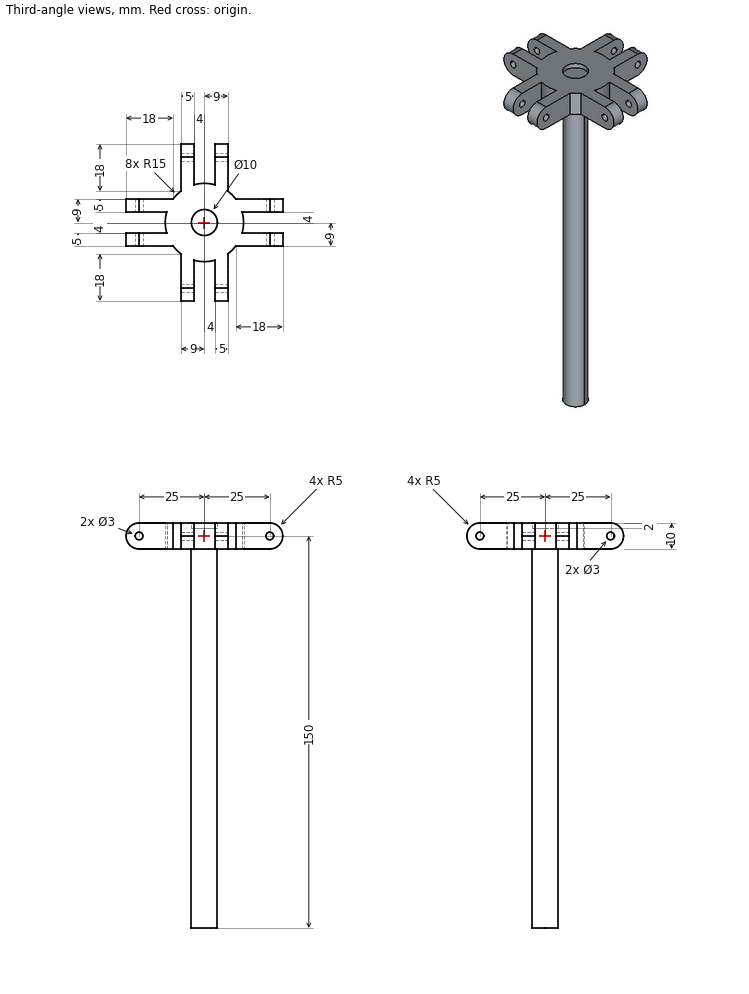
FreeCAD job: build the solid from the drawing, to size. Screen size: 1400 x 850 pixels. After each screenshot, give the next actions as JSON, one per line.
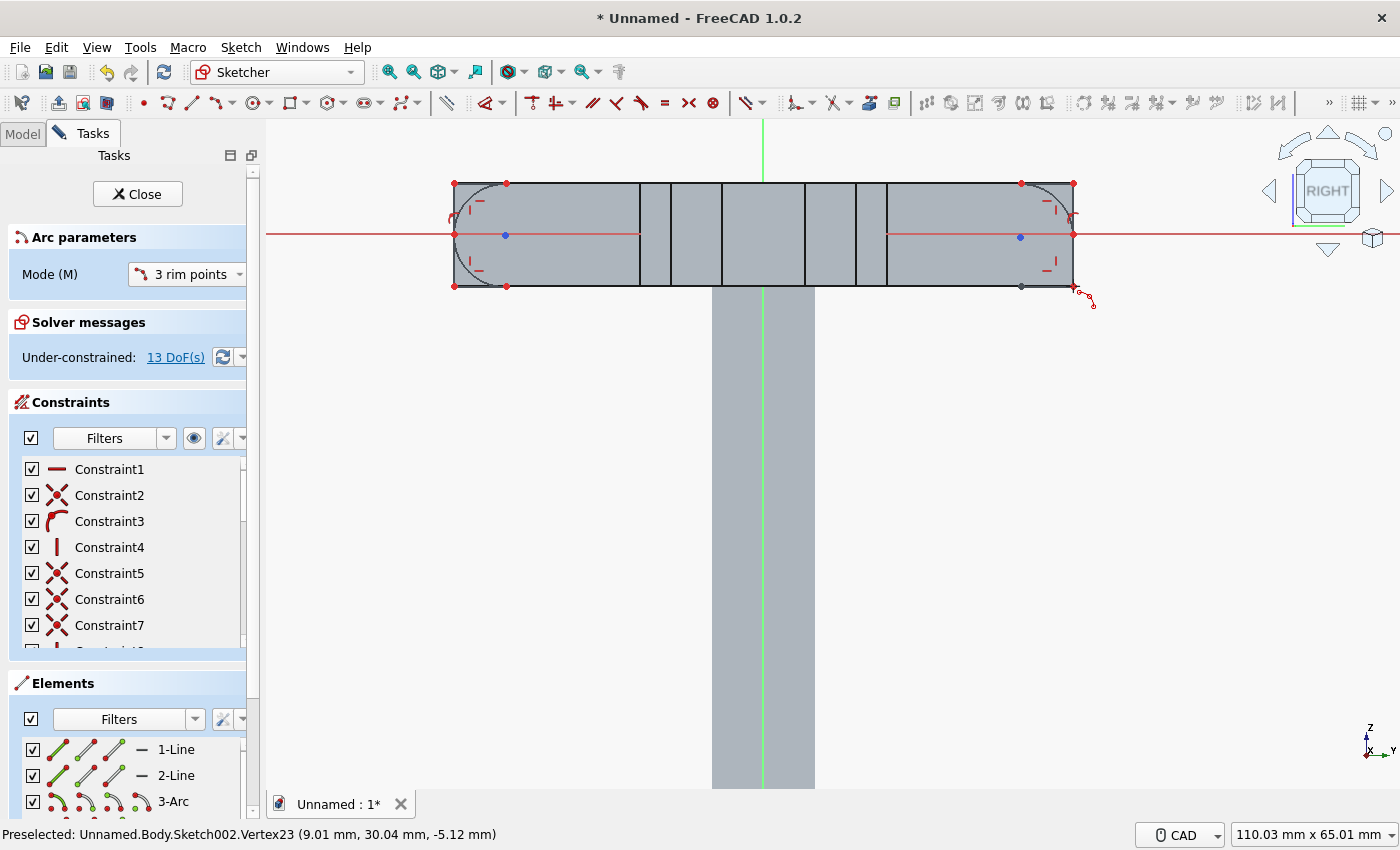
{"action": "left_click", "coordinate": [1073, 234]}
{"action": "left_click", "coordinate": [1021, 287]}
{"action": "left_click", "coordinate": [1057, 271]}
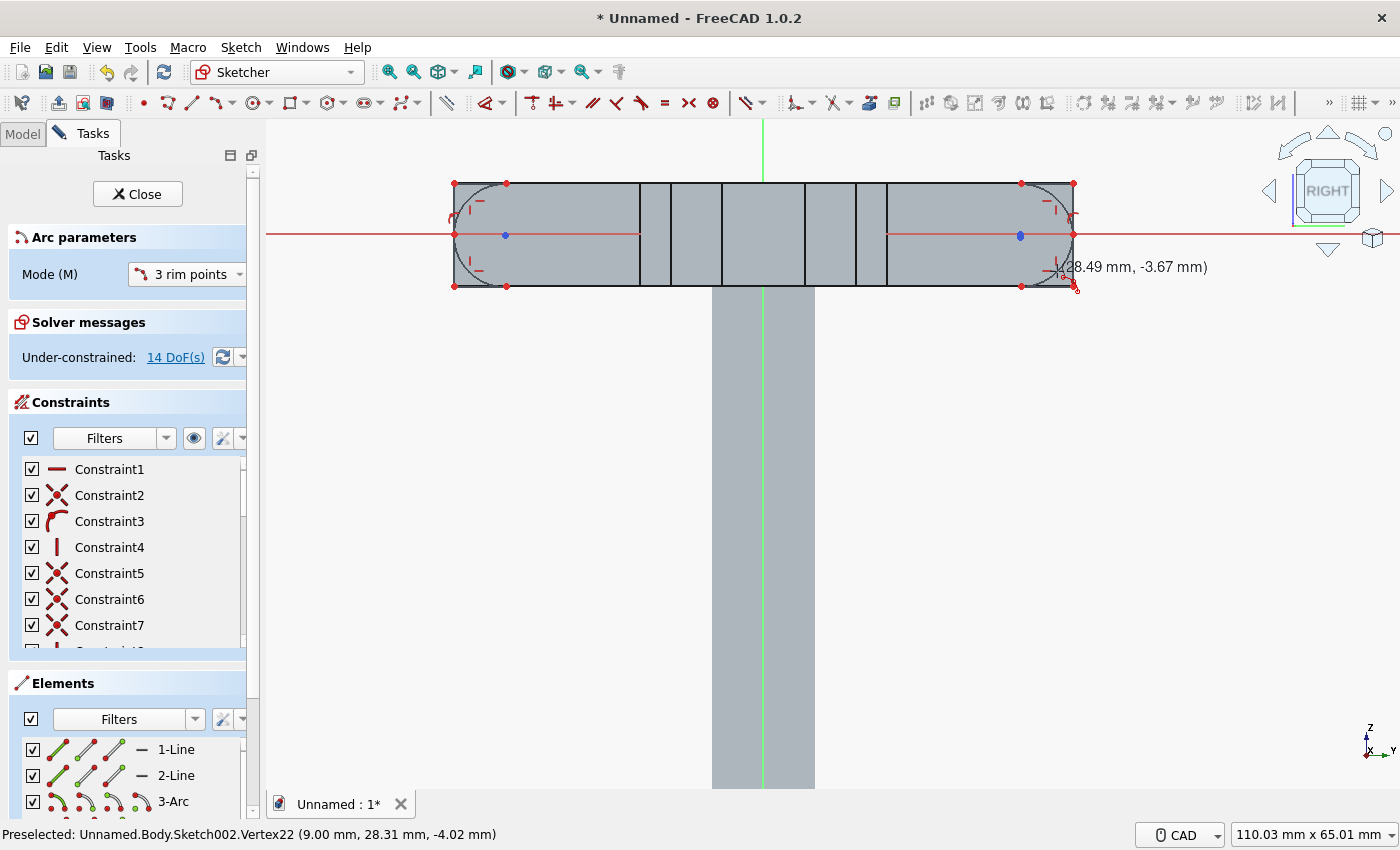
{"action": "key", "text": "g c"}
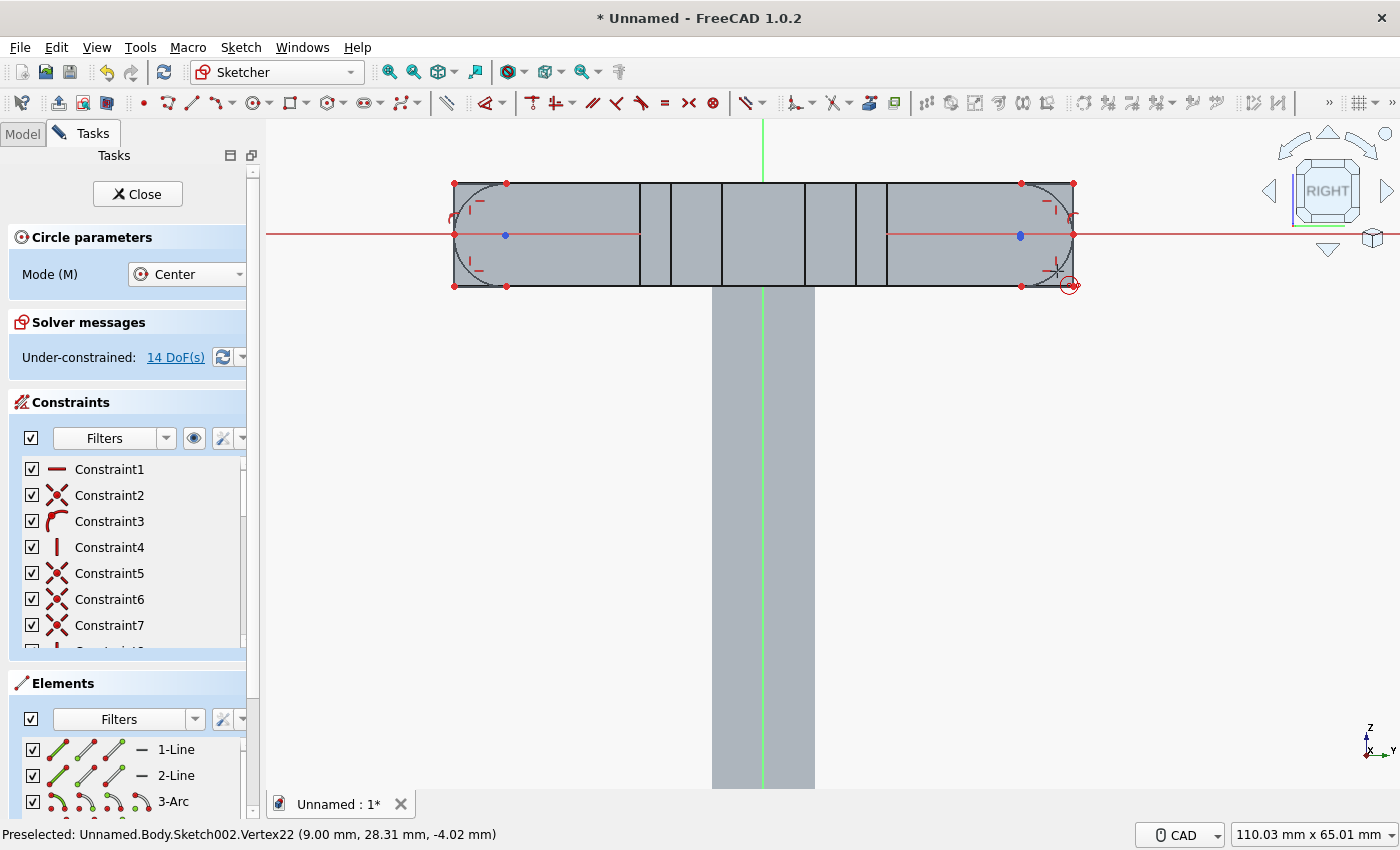
{"action": "scroll", "coordinate": [1021, 234], "scroll_direction": "up", "scroll_amount": 2}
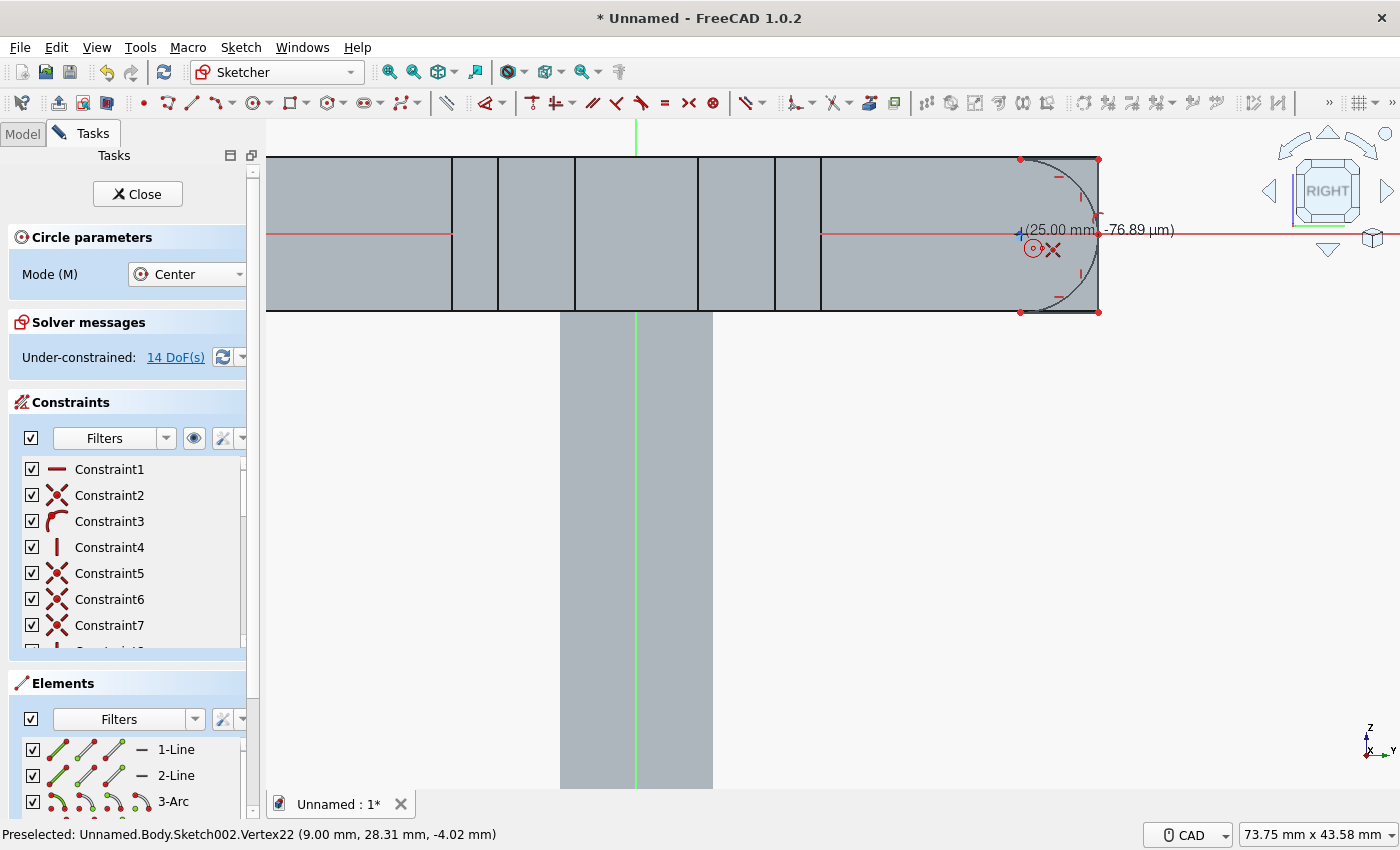
{"action": "left_click", "coordinate": [1021, 234]}
{"action": "mouse_move", "coordinate": [1037, 218]}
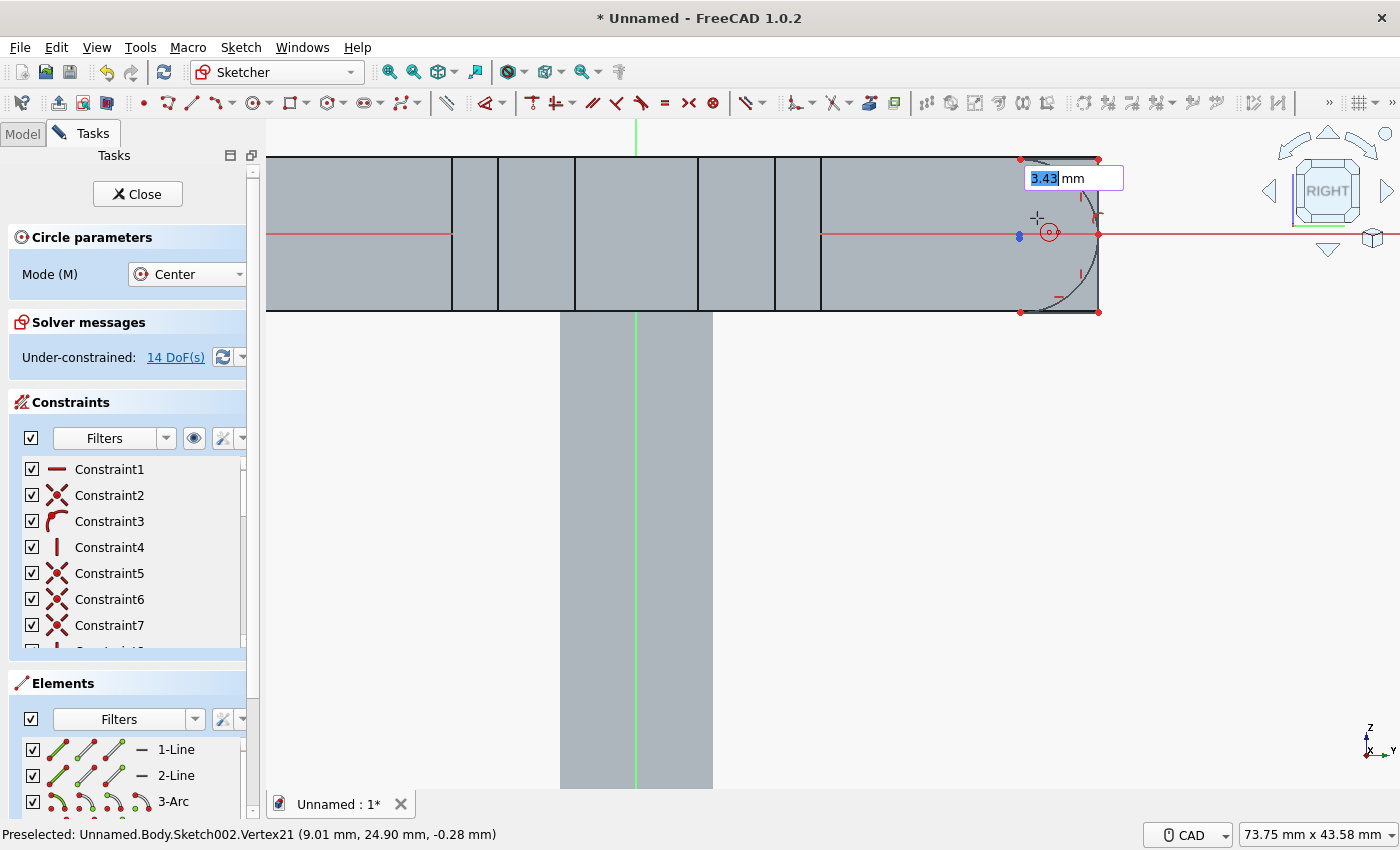
{"action": "type", "text": "3"}
{"action": "key", "text": "Return"}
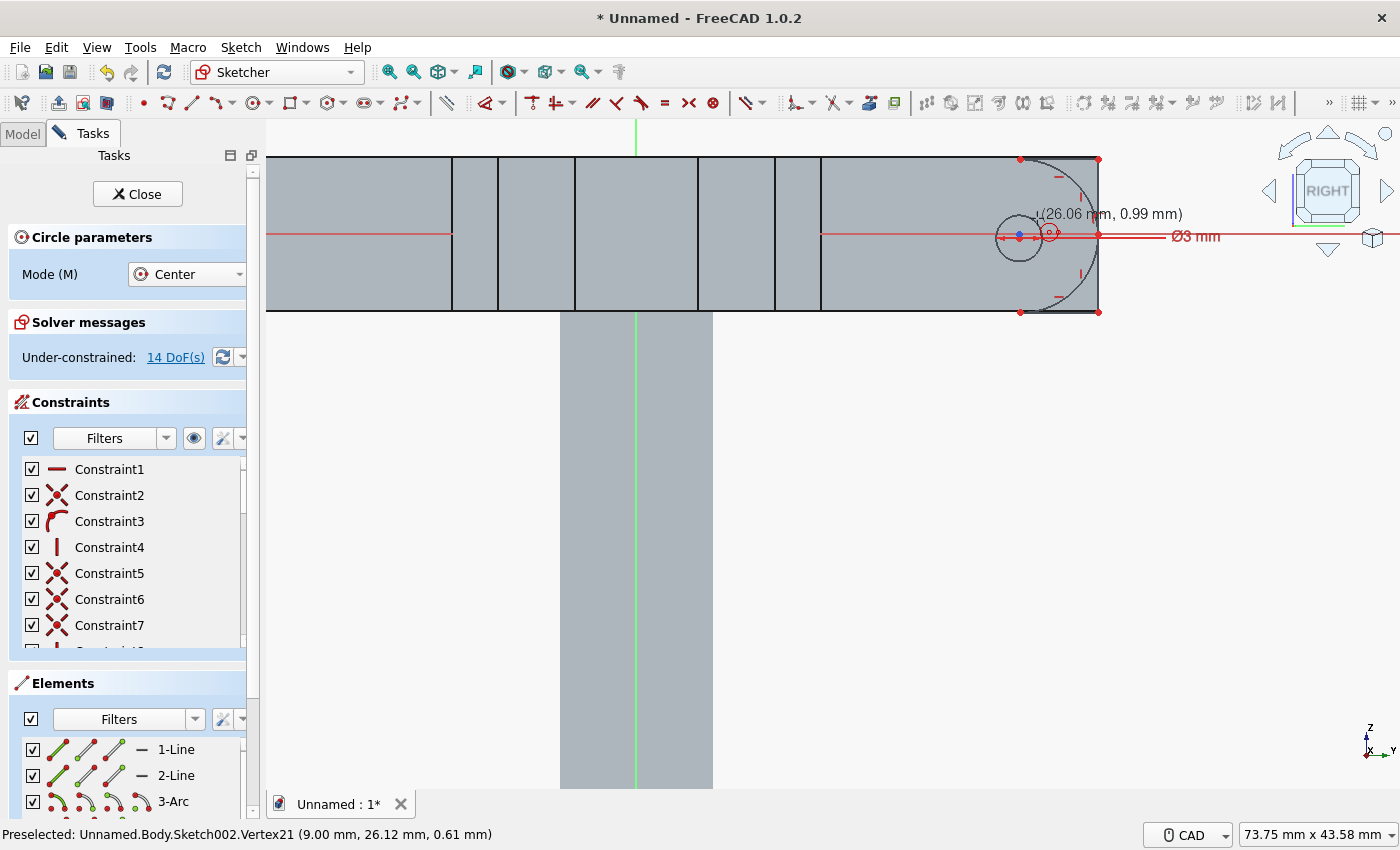
{"action": "scroll", "coordinate": [1025, 761], "scroll_direction": "down", "scroll_amount": 2}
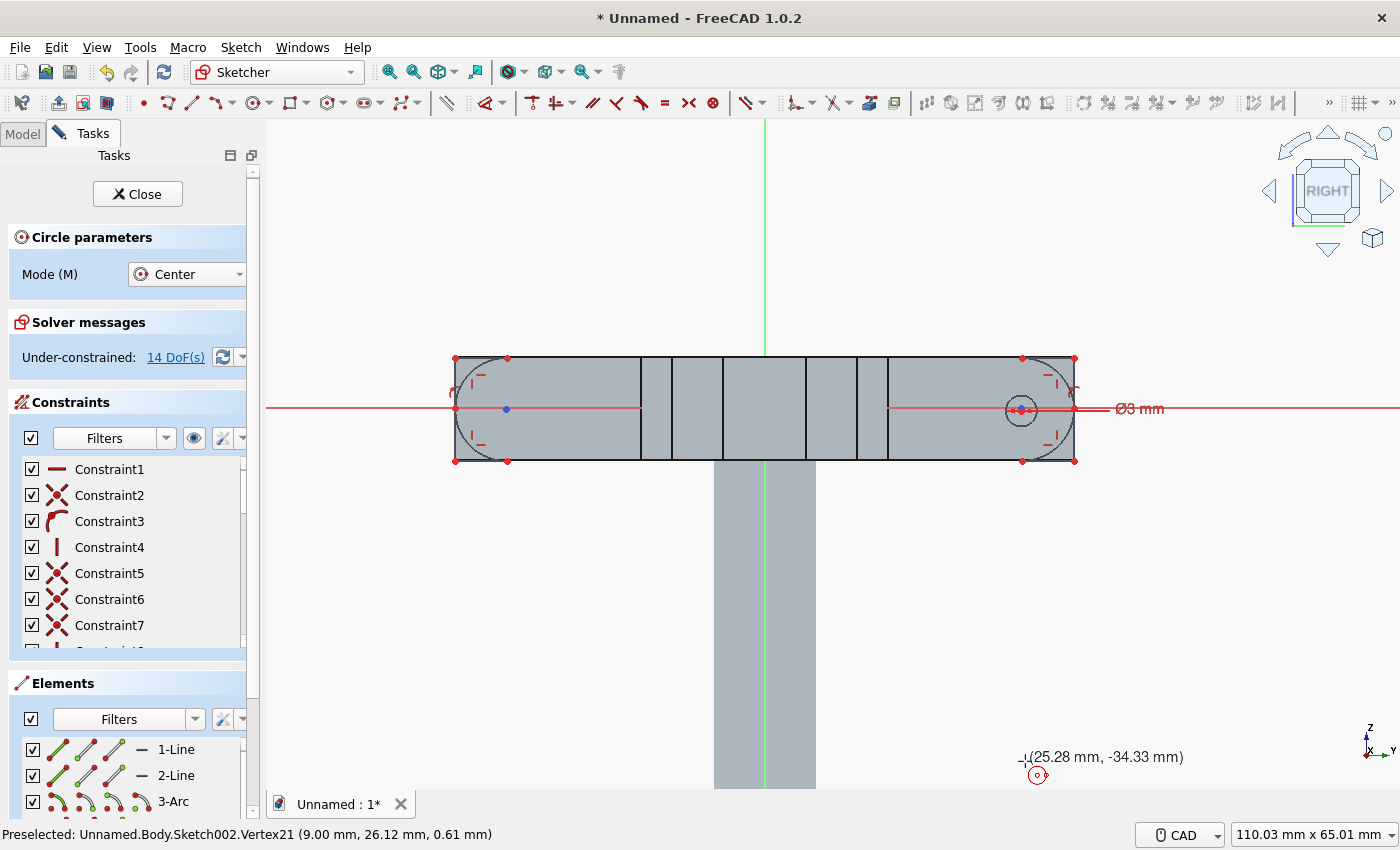
{"action": "scroll", "coordinate": [507, 408], "scroll_direction": "up", "scroll_amount": 2}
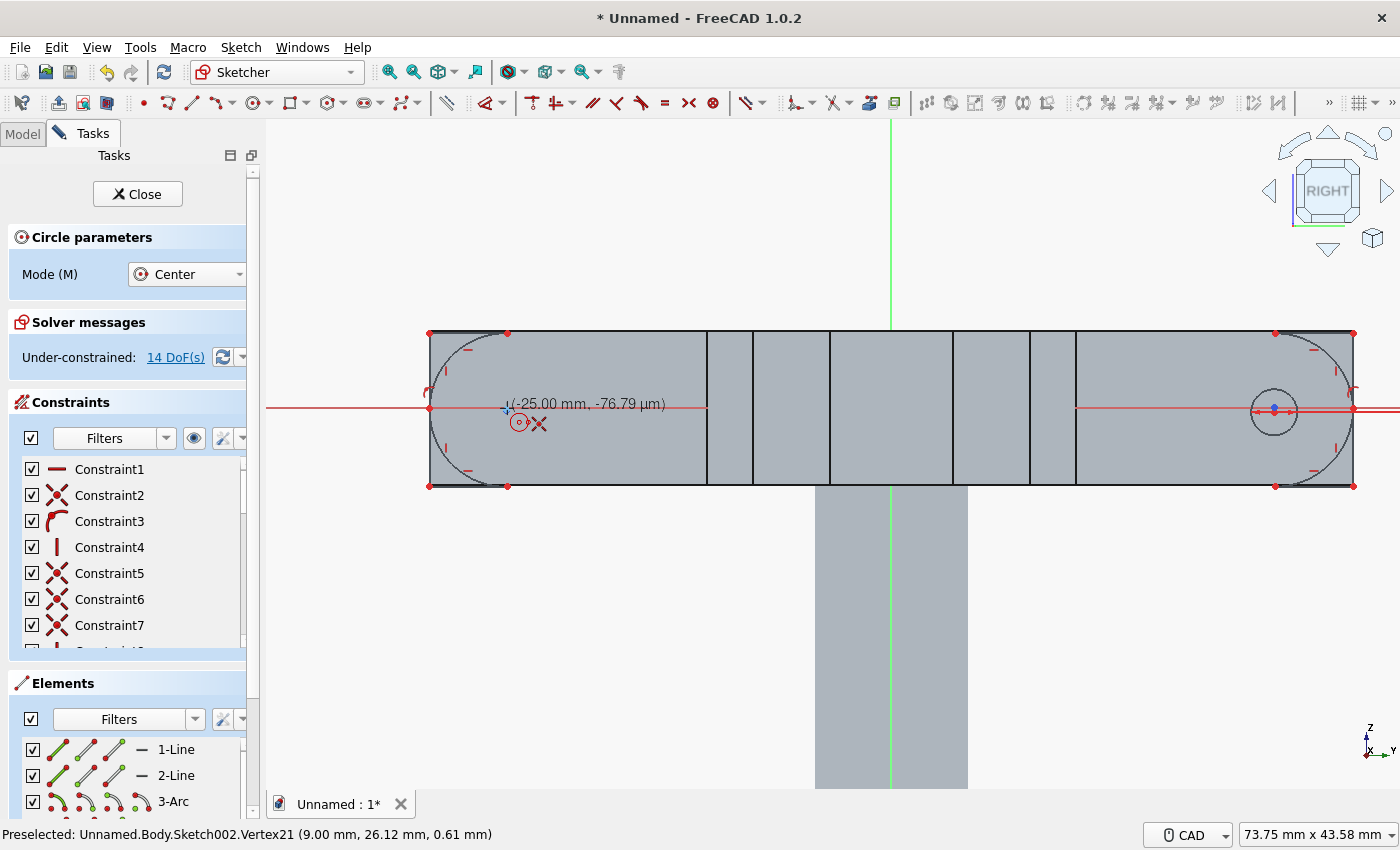
{"action": "left_click", "coordinate": [507, 408]}
{"action": "mouse_move", "coordinate": [523, 392]}